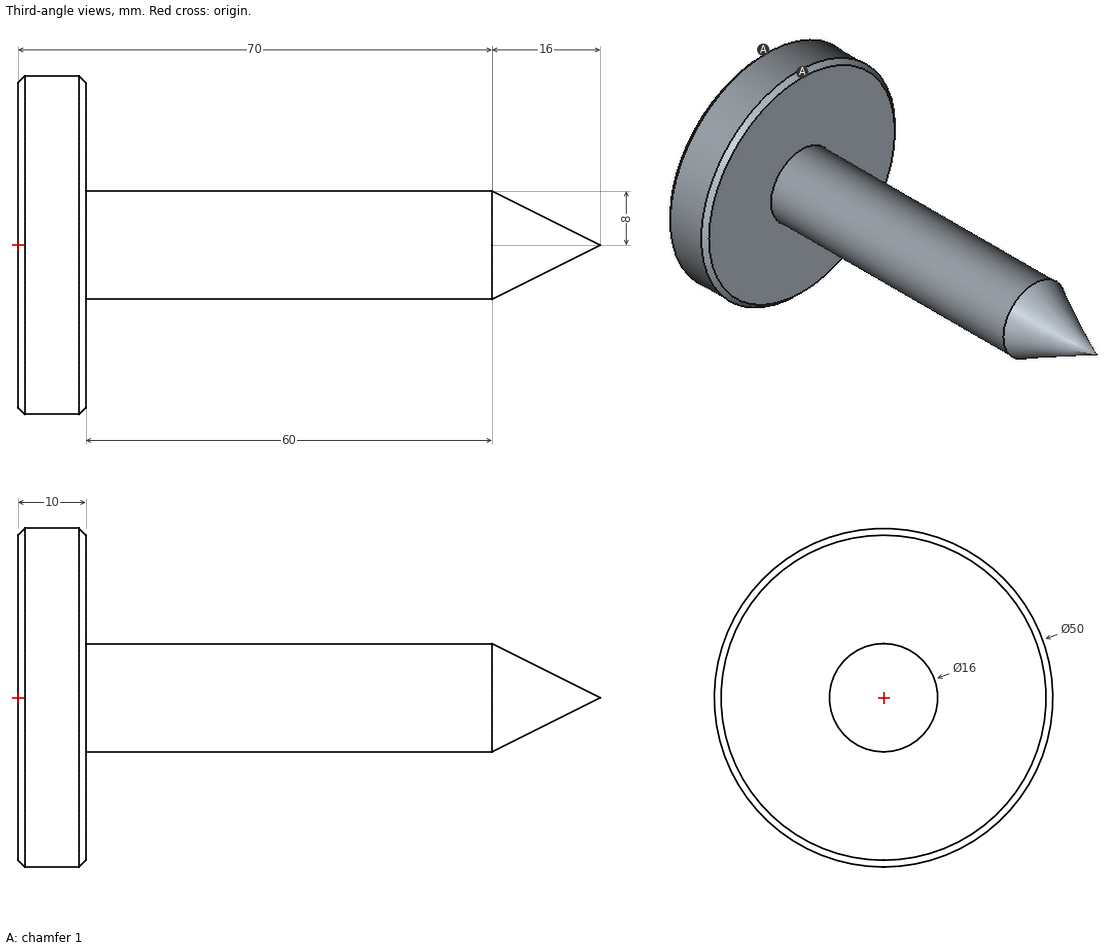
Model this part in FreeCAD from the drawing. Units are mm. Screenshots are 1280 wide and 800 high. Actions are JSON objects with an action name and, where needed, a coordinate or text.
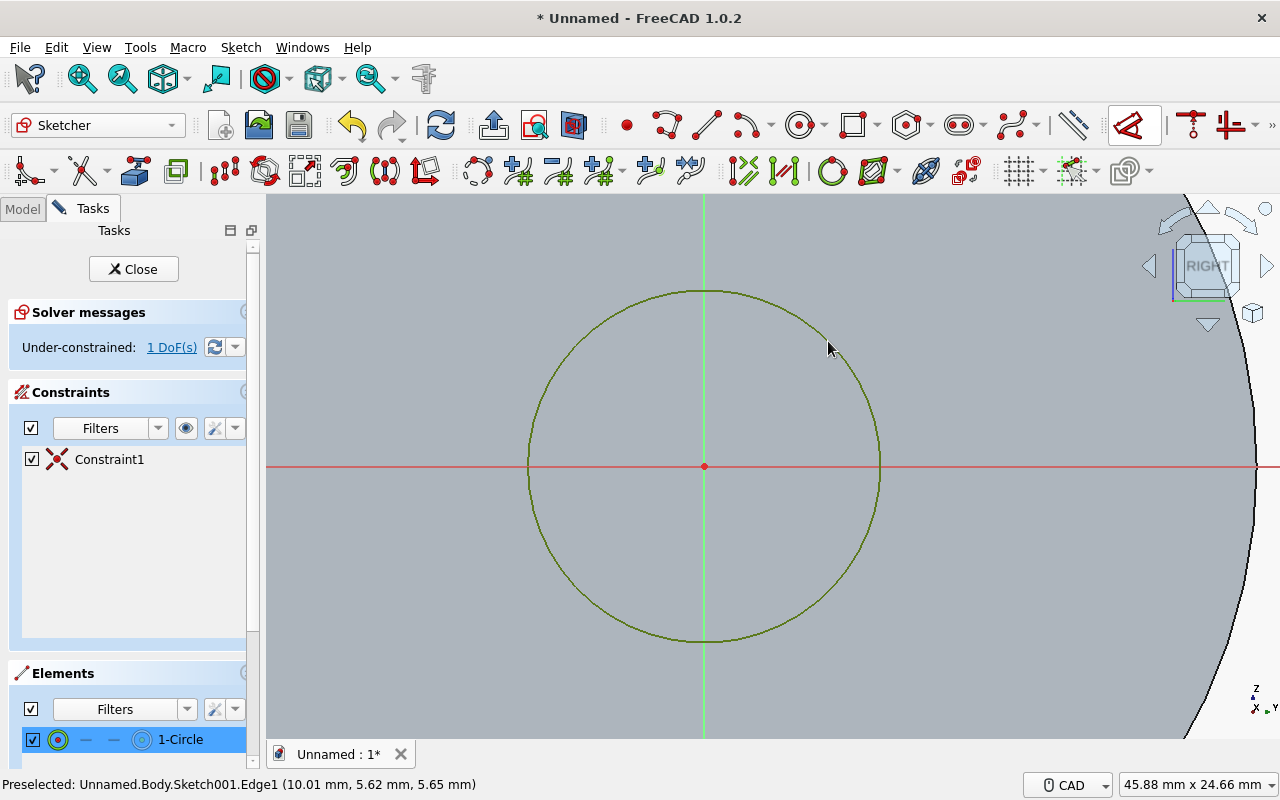
{"action": "key", "text": "k o"}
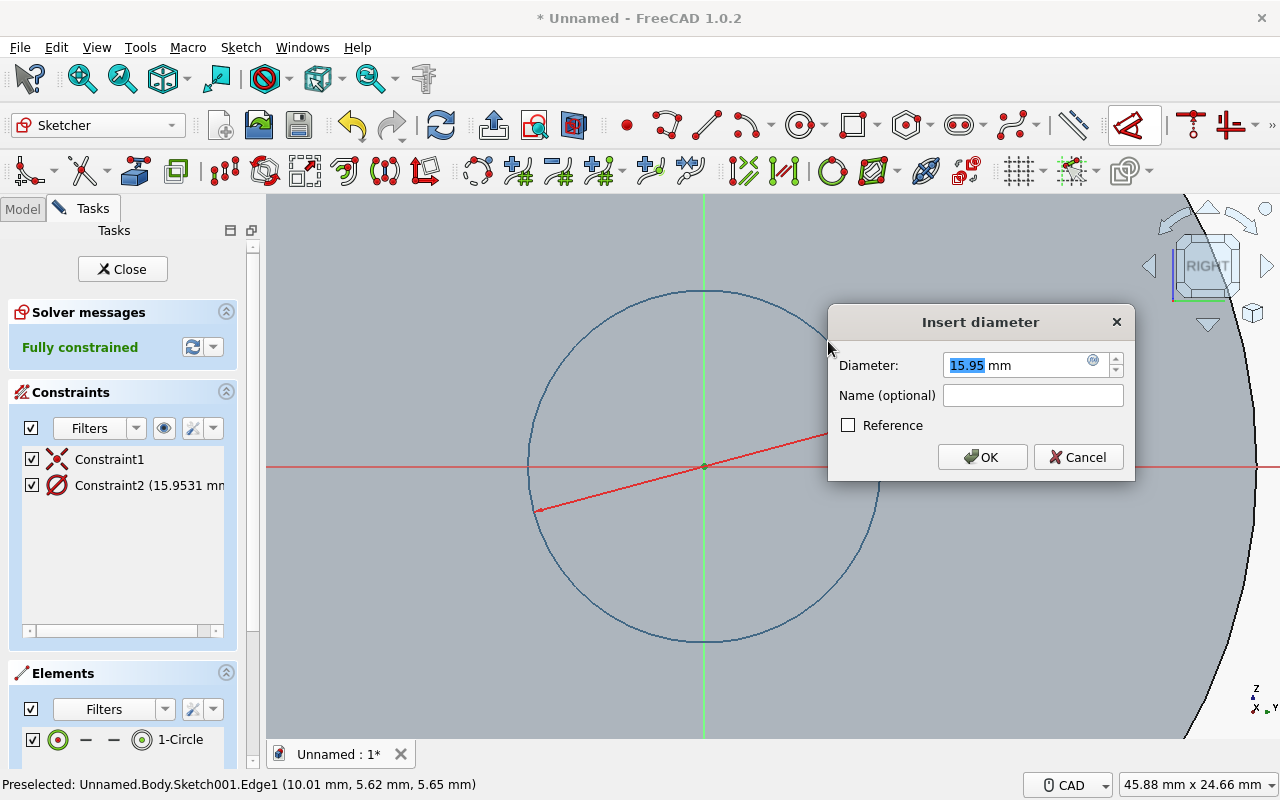
{"action": "type", "text": "16"}
{"action": "key", "text": "Return"}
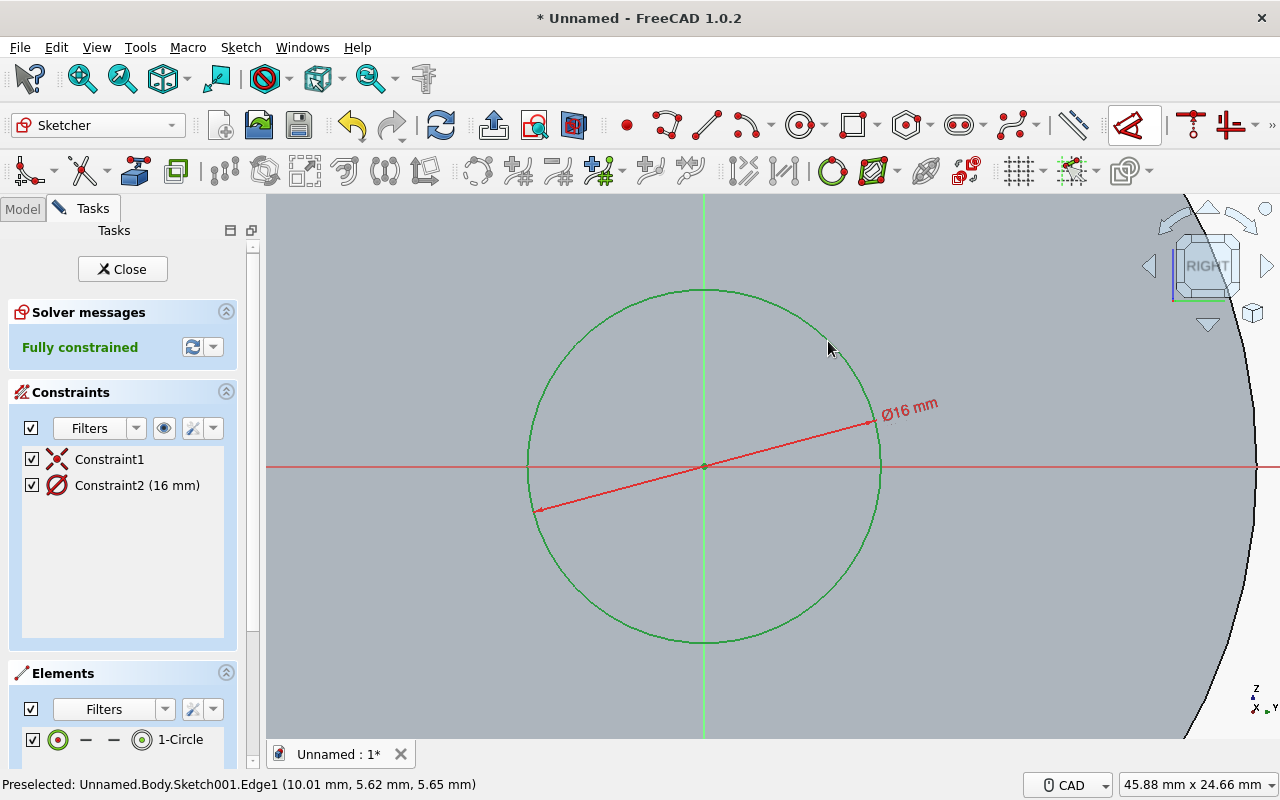
{"action": "left_click", "coordinate": [123, 269]}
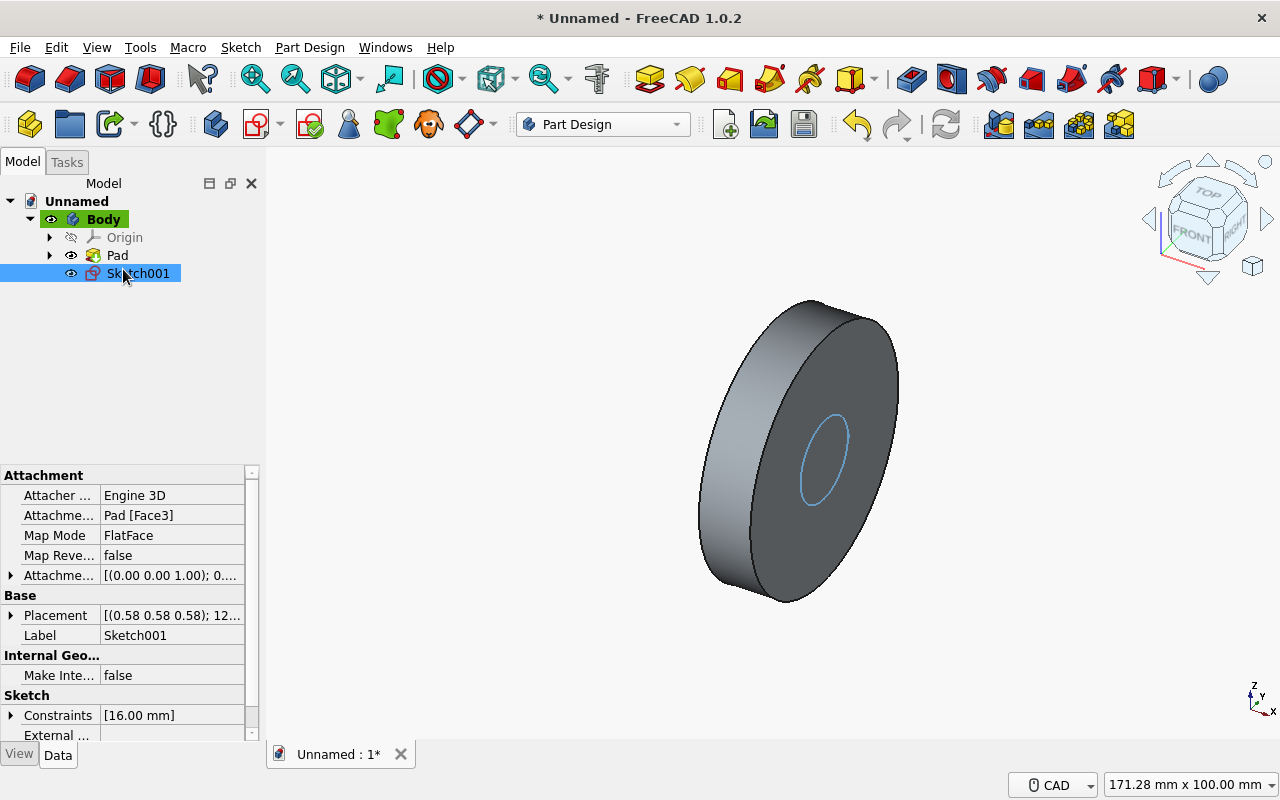
{"action": "left_click", "coordinate": [650, 80]}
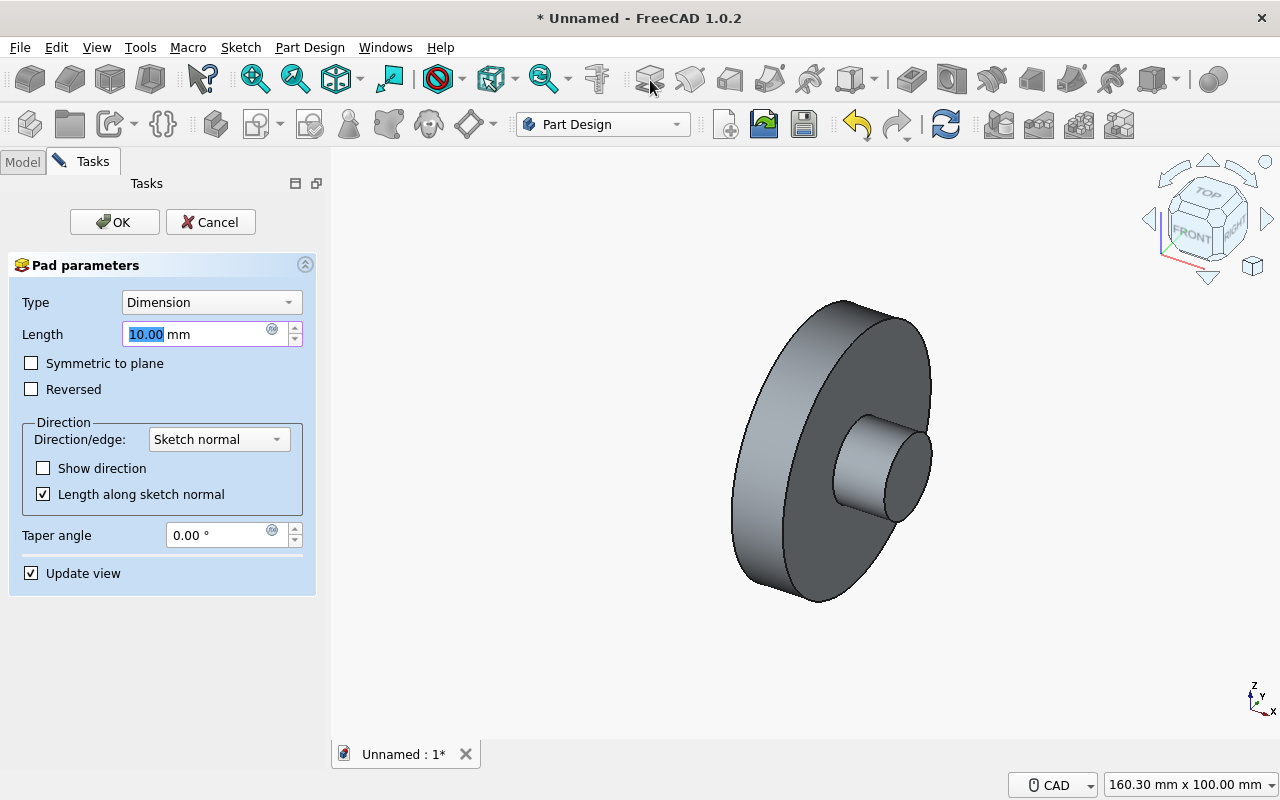
{"action": "type", "text": "60"}
{"action": "key", "text": "Tab"}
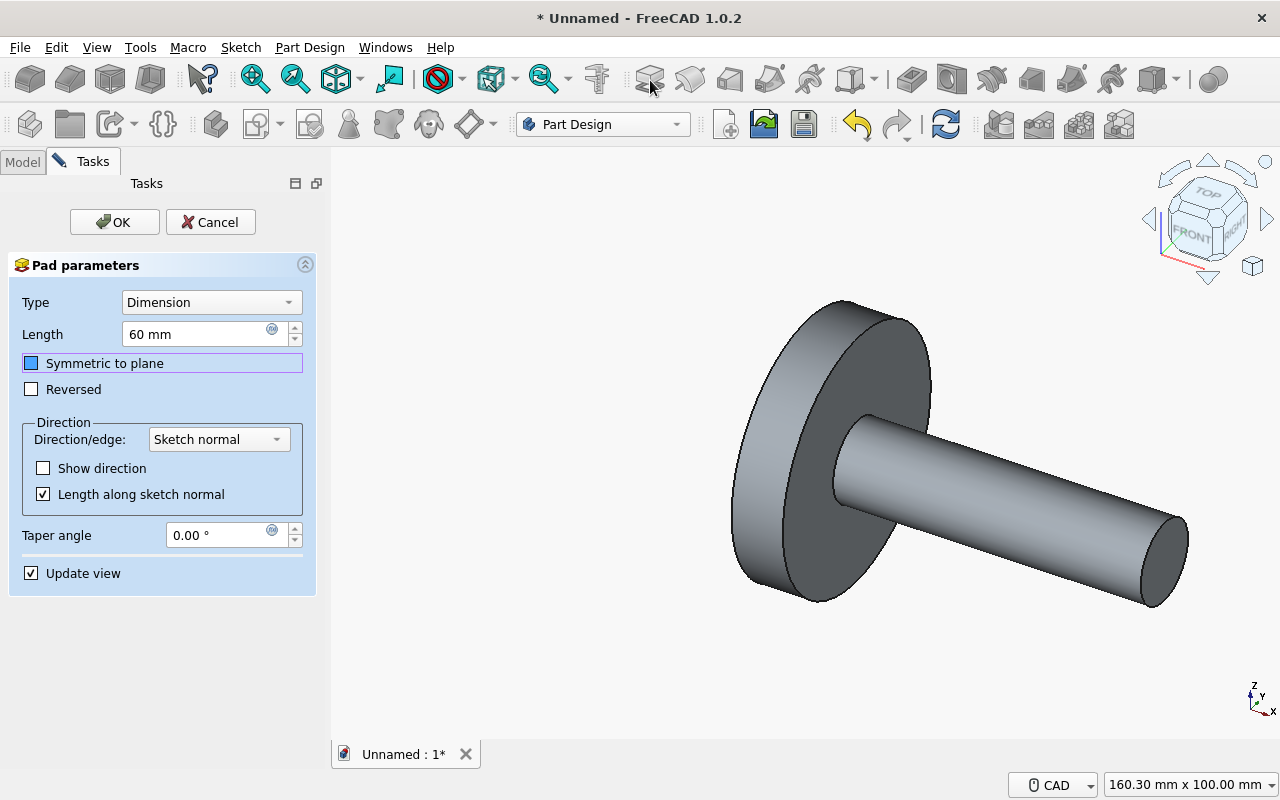
{"action": "left_click", "coordinate": [115, 222]}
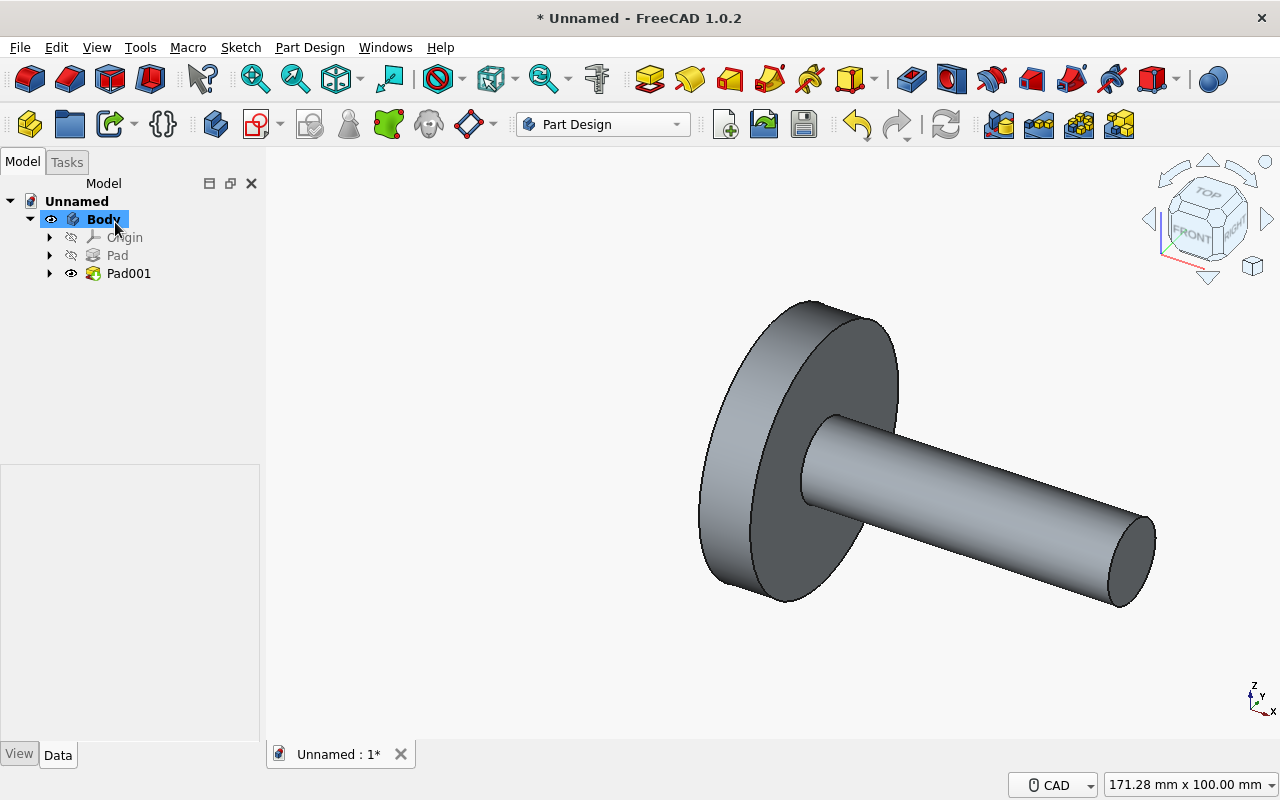
{"action": "key", "text": "v f"}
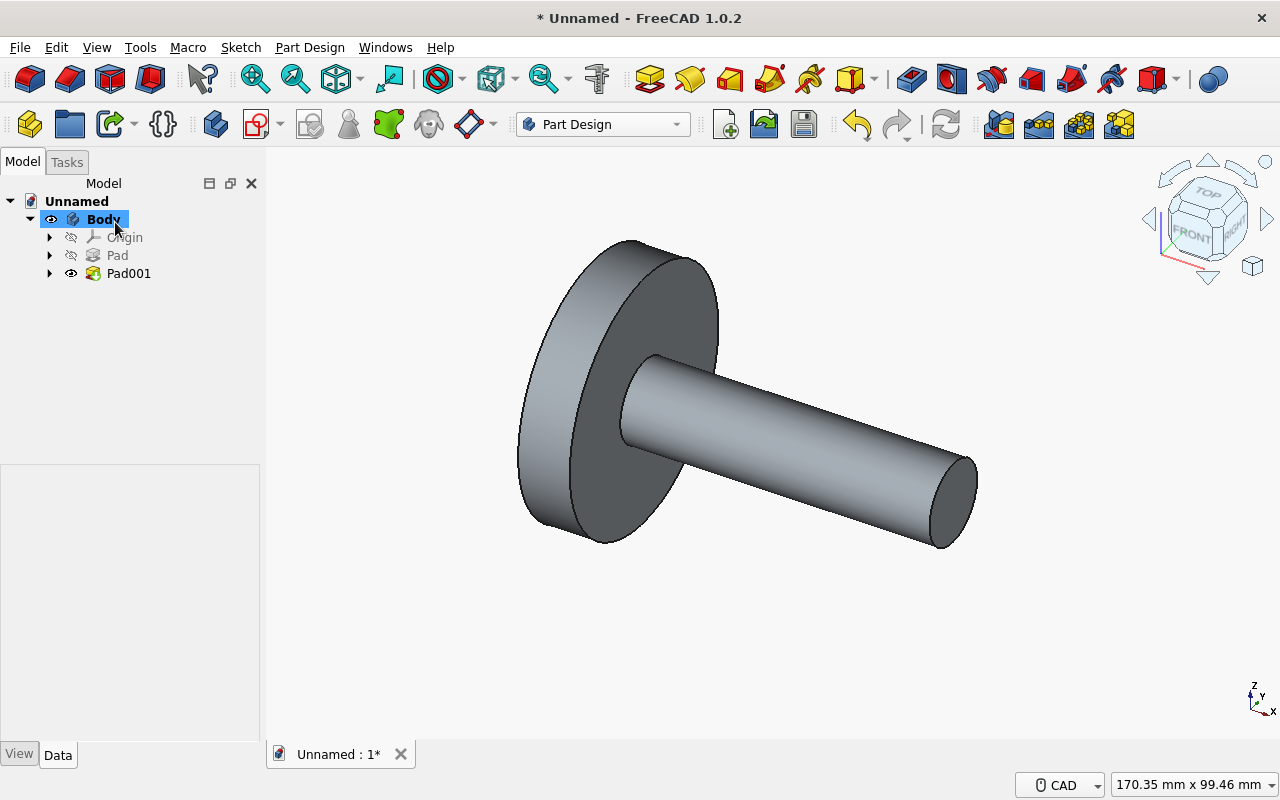
{"action": "left_click", "coordinate": [256, 124]}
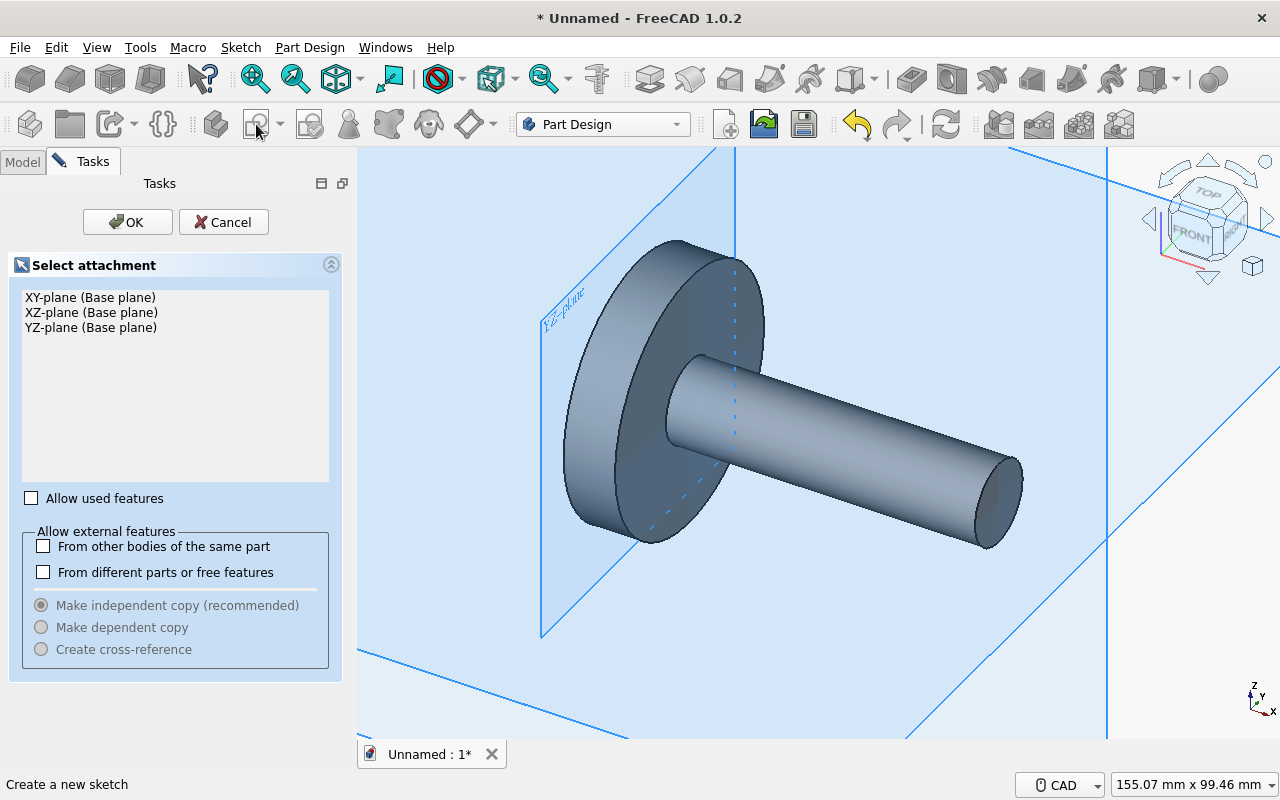
{"action": "left_click", "coordinate": [82, 298]}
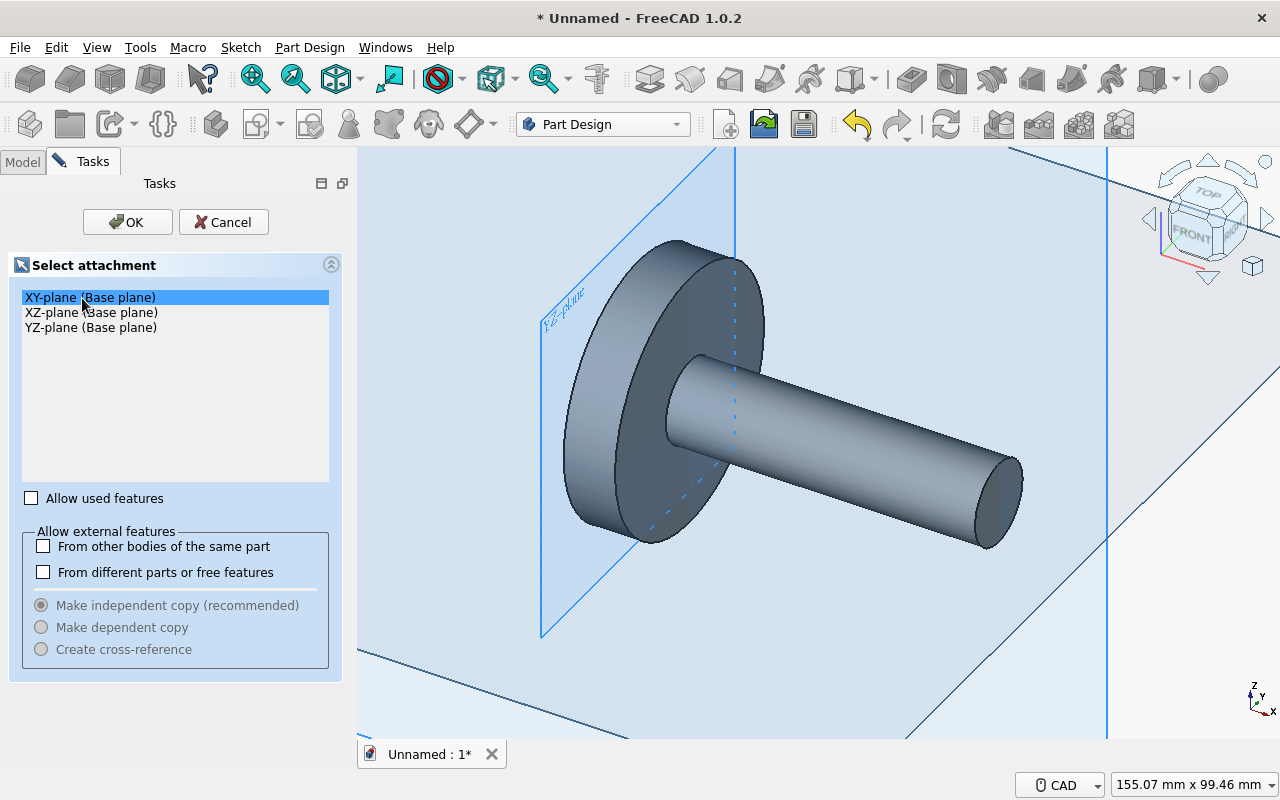
{"action": "left_click", "coordinate": [128, 222]}